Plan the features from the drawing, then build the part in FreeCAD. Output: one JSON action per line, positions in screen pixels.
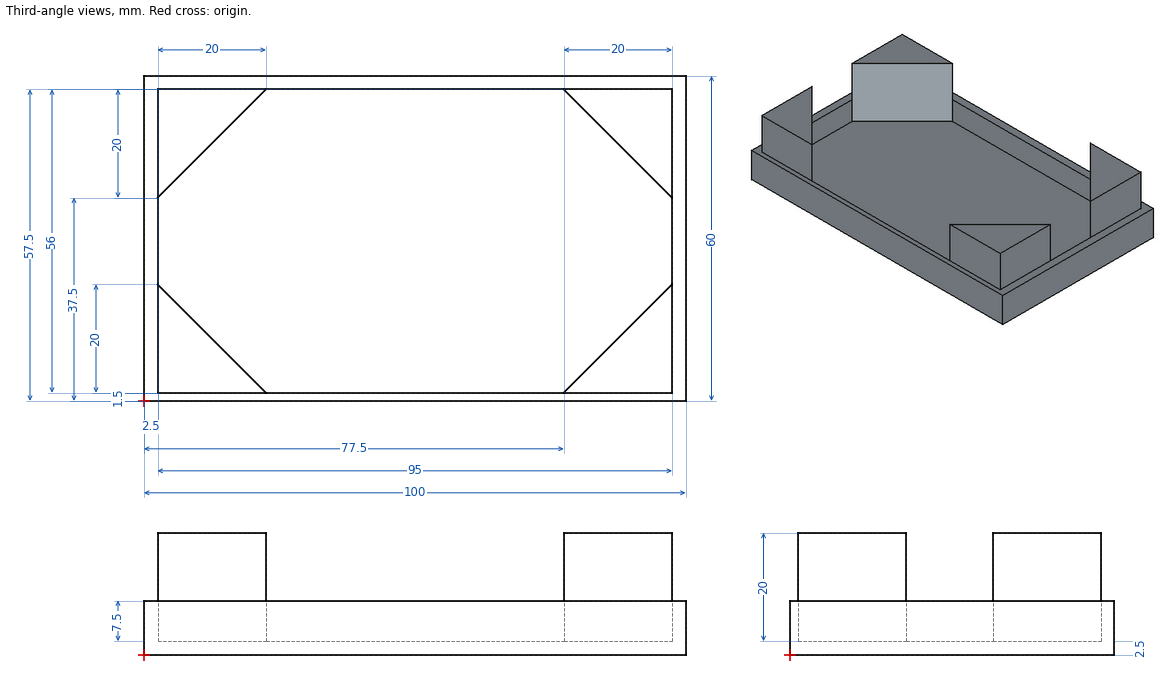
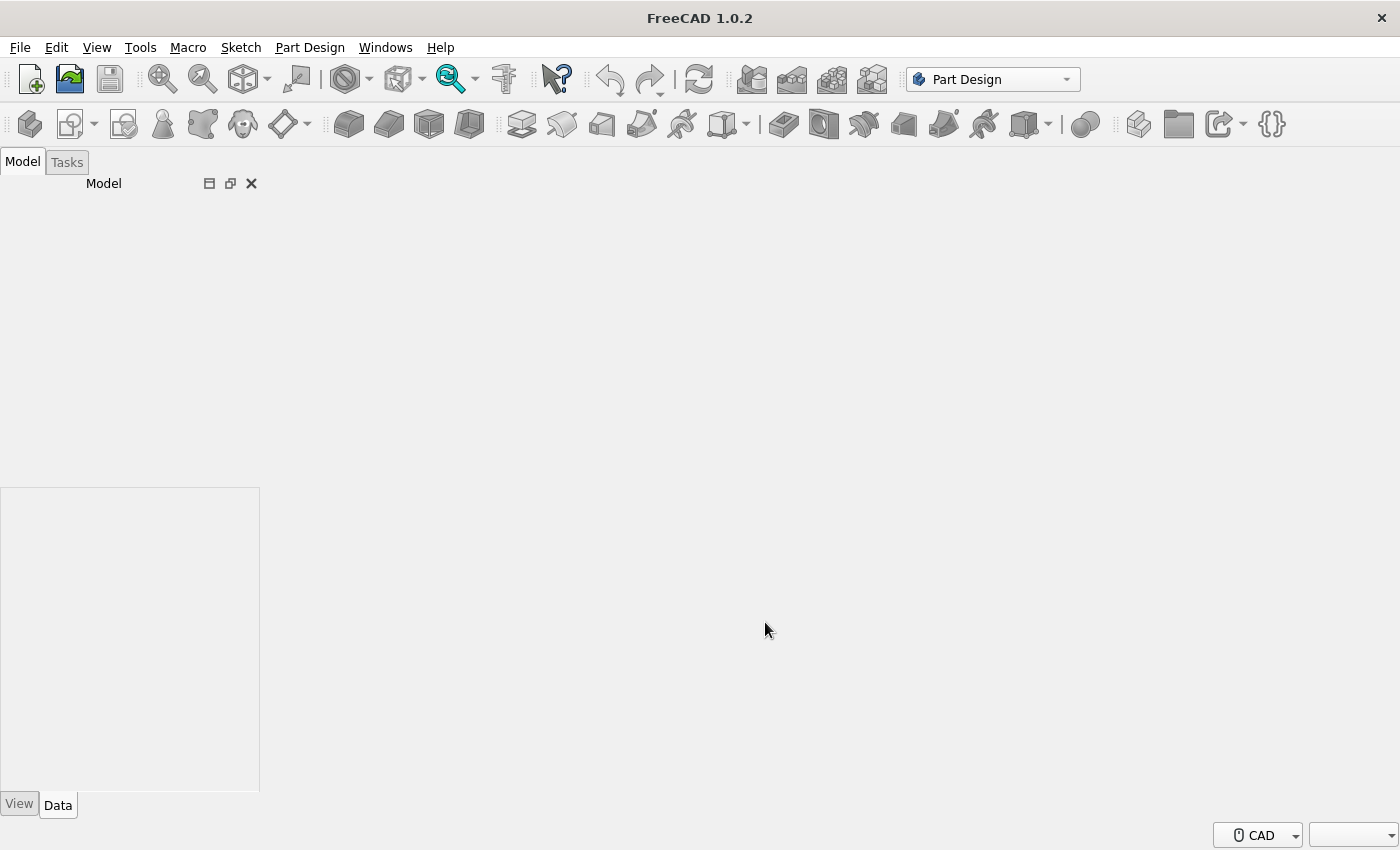
{"action": "left_click", "coordinate": [30, 80]}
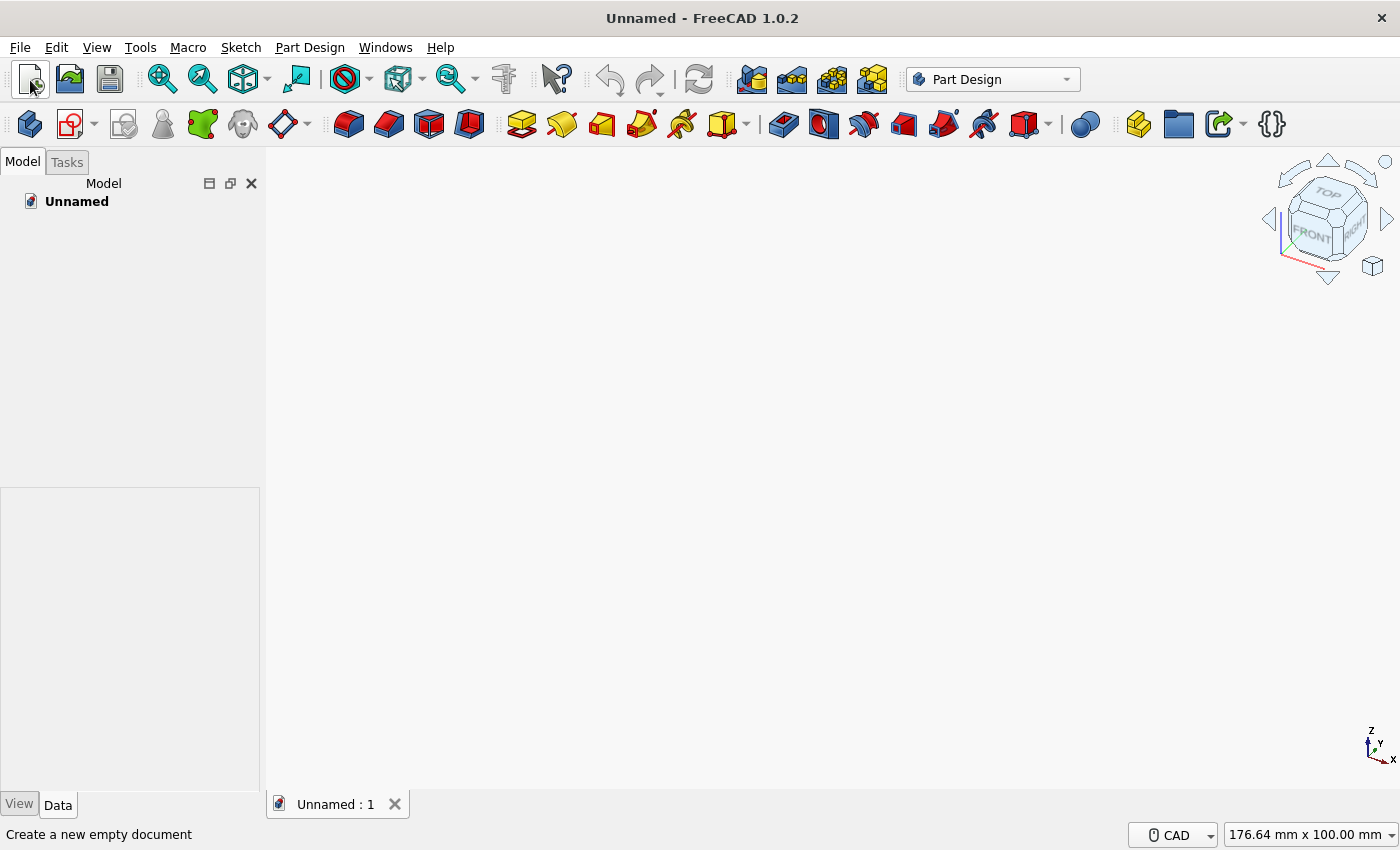
{"action": "left_click", "coordinate": [70, 124]}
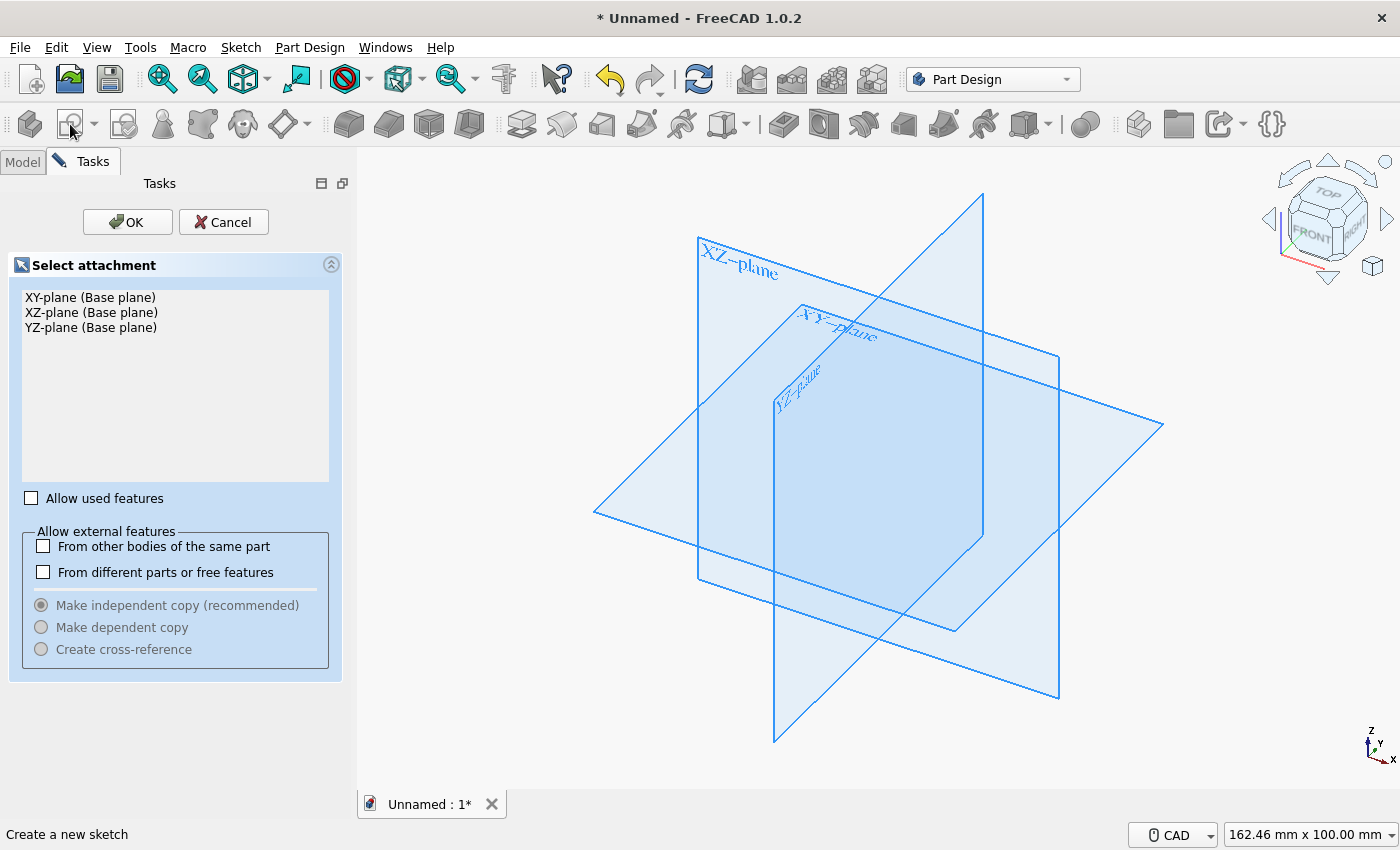
{"action": "left_click", "coordinate": [82, 298]}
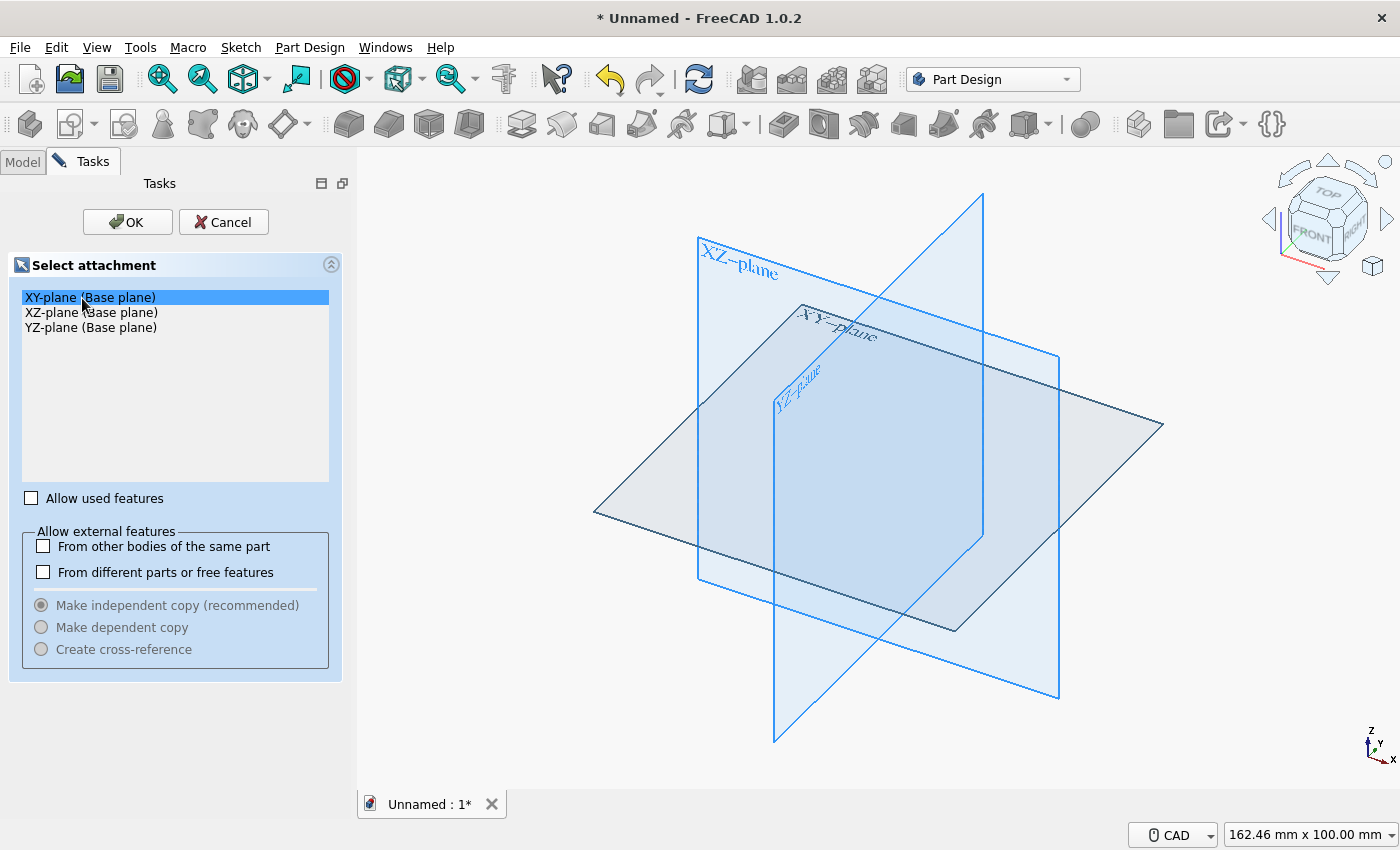
{"action": "left_click", "coordinate": [128, 222]}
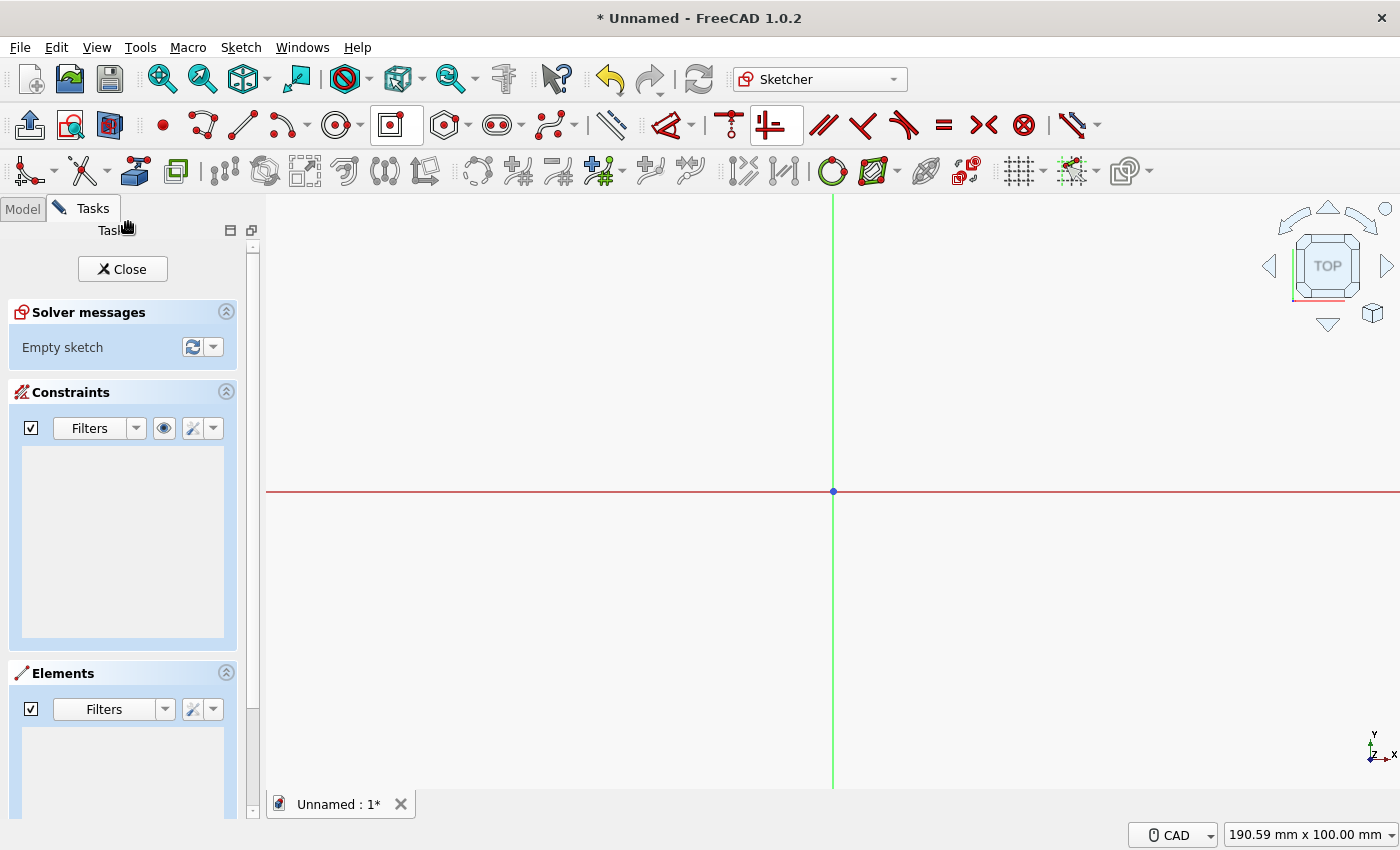
{"action": "scroll", "coordinate": [294, 761], "scroll_direction": "down", "scroll_amount": 2}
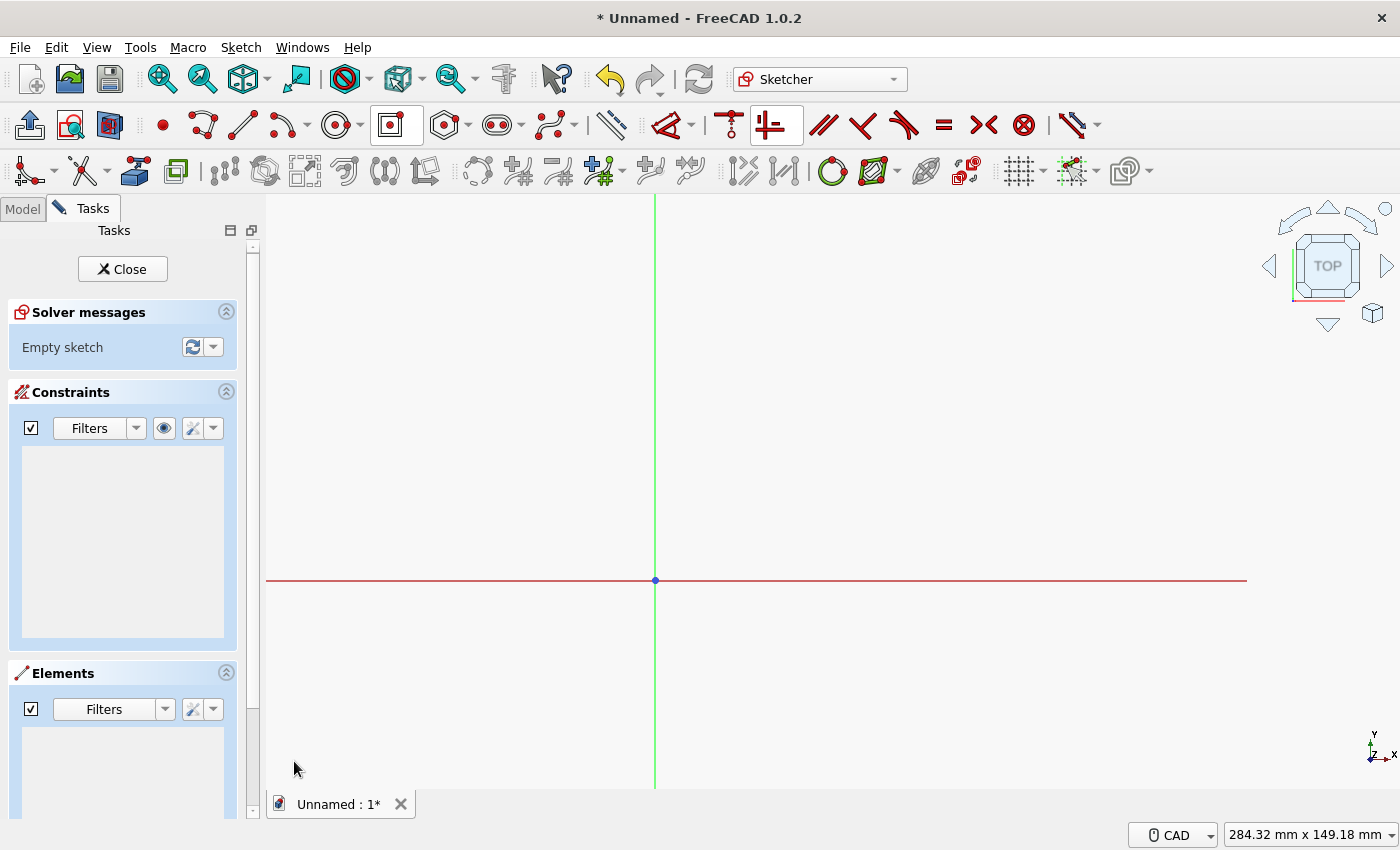
{"action": "scroll", "coordinate": [1038, 399], "scroll_direction": "up", "scroll_amount": 2}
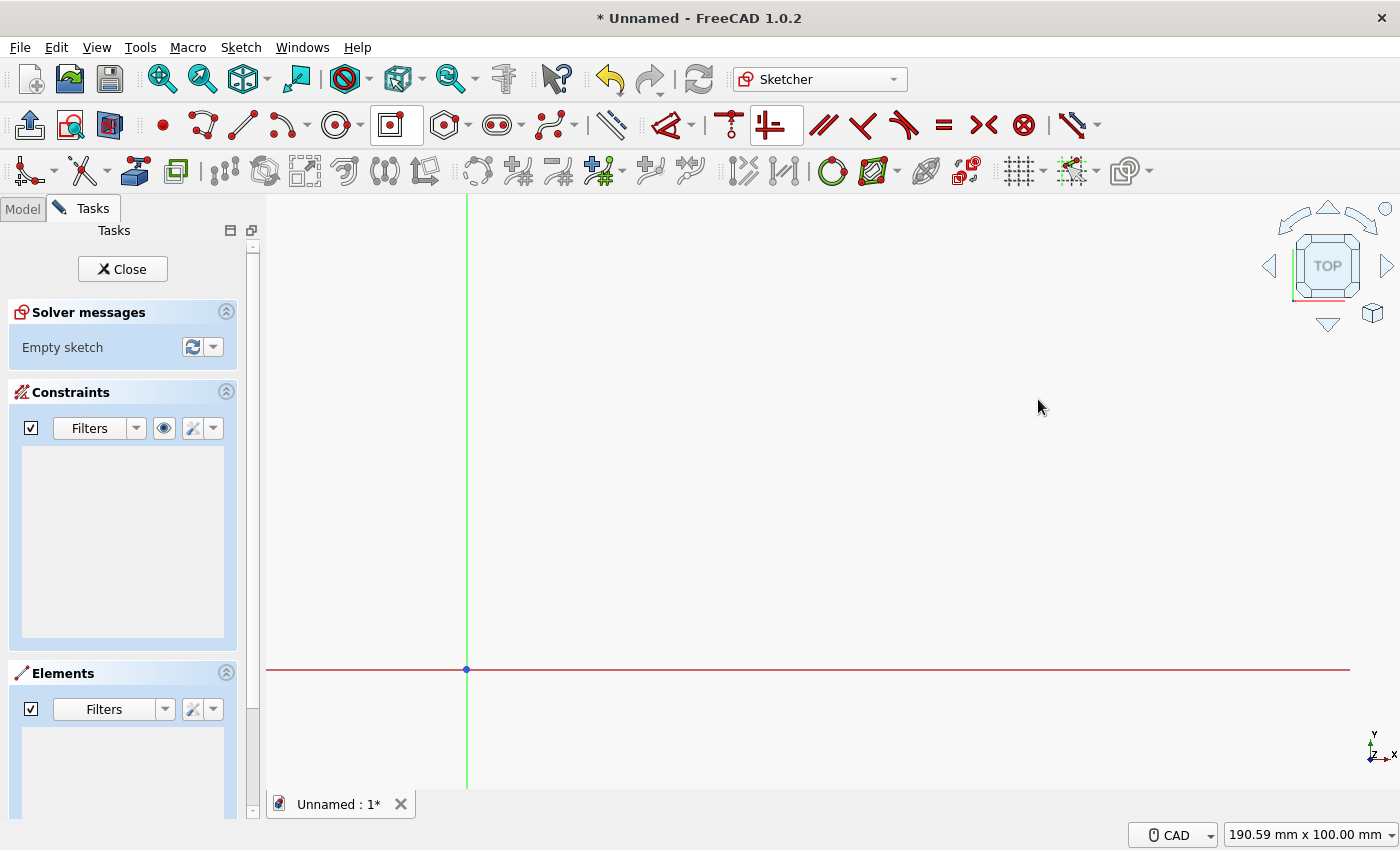
{"action": "left_click", "coordinate": [418, 126]}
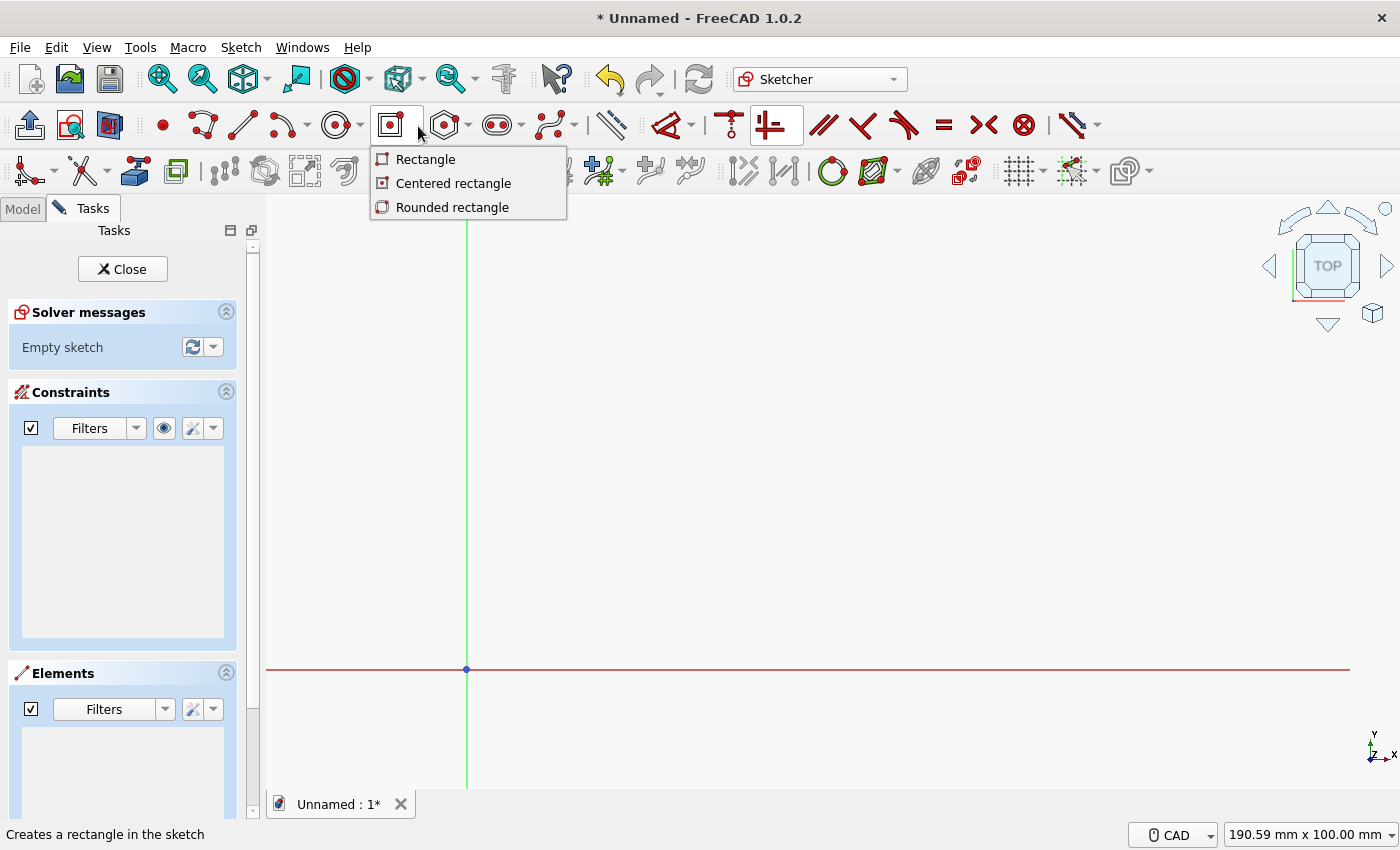
{"action": "left_click", "coordinate": [468, 159]}